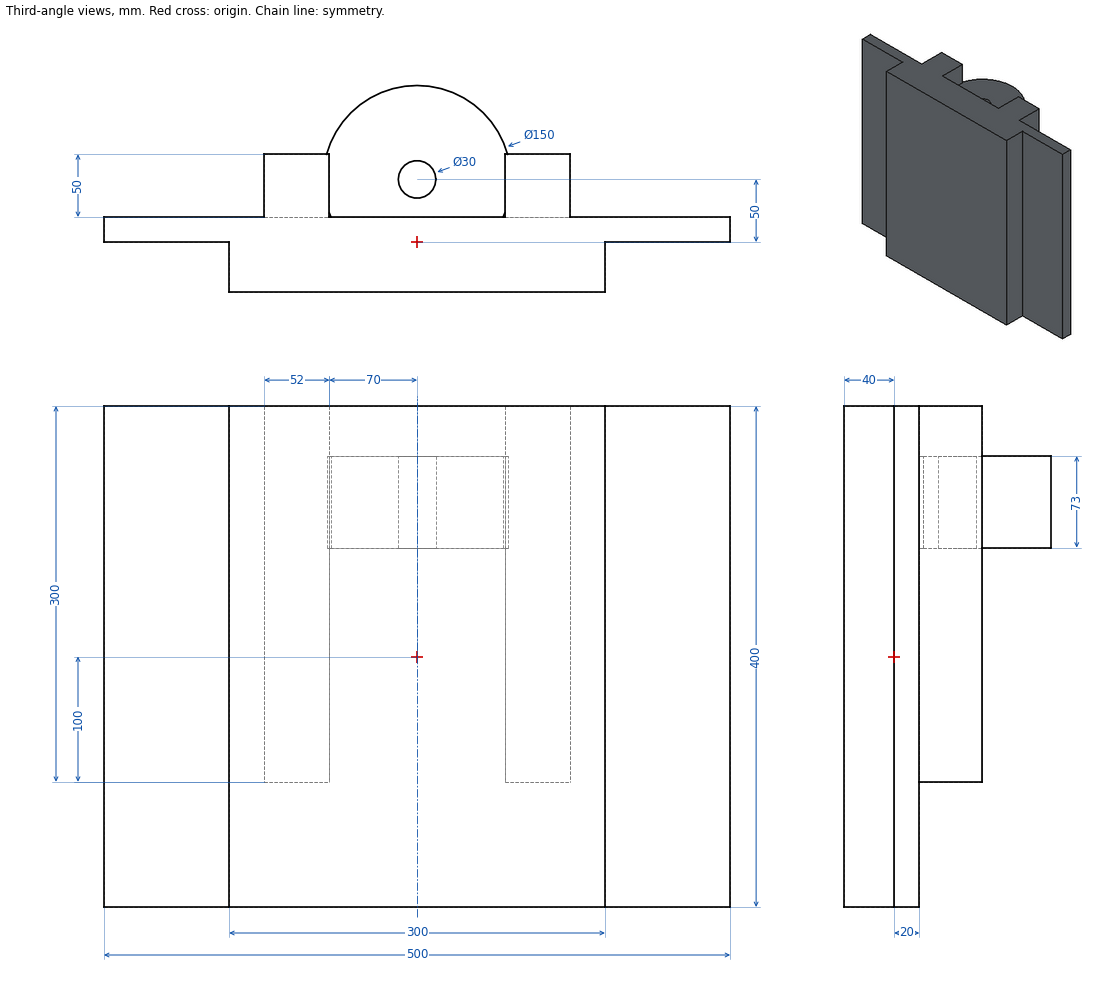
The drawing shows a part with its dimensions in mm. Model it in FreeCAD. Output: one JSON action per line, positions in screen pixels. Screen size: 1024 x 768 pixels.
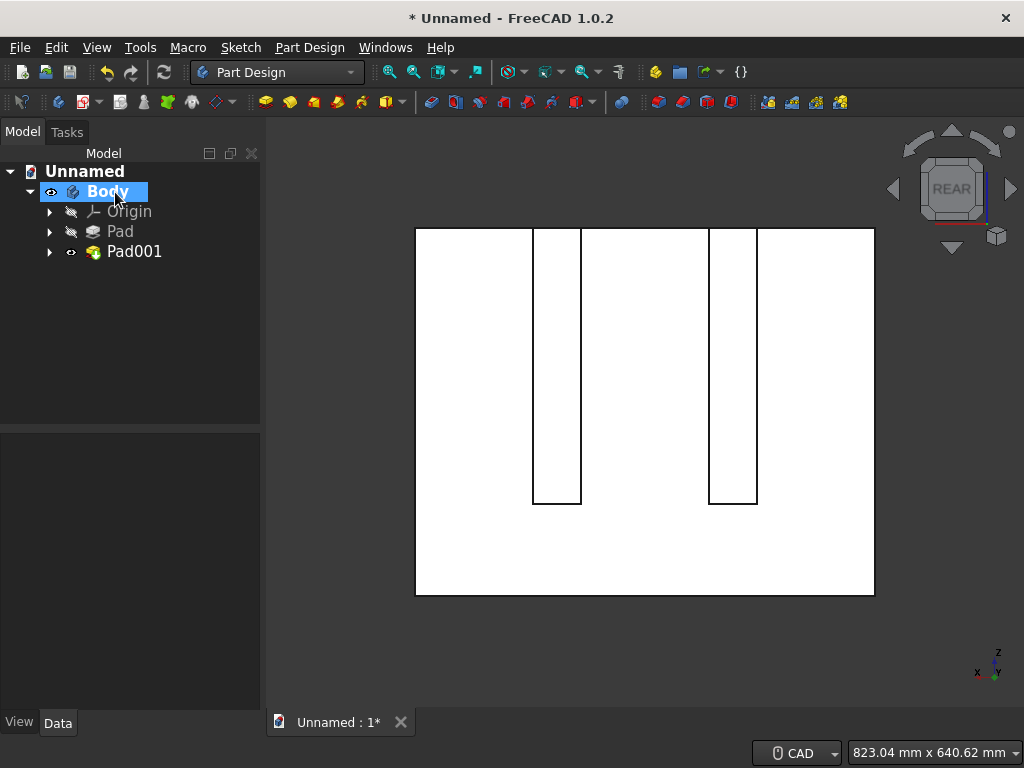
{"action": "left_click", "coordinate": [84, 102]}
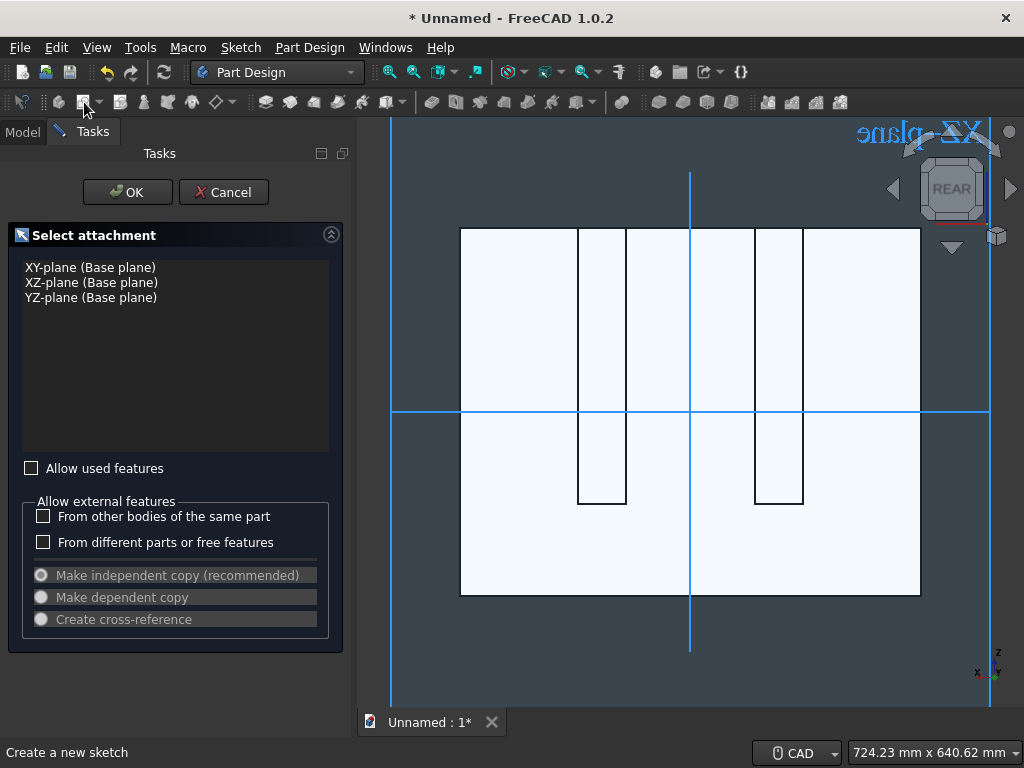
{"action": "left_click", "coordinate": [82, 282]}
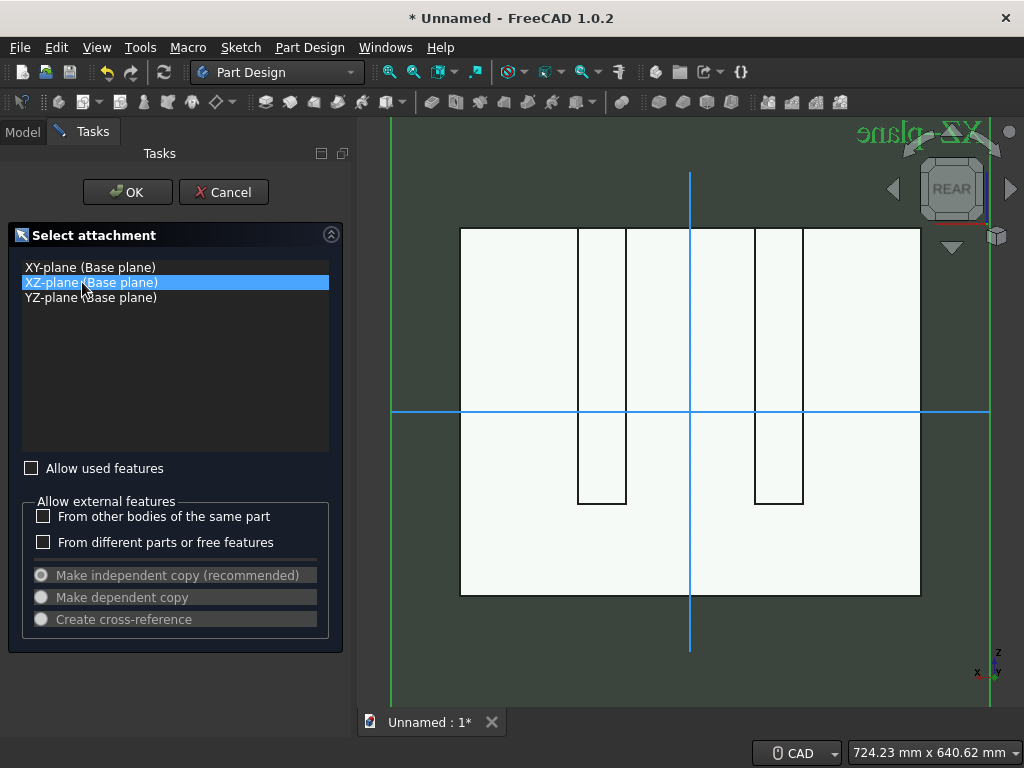
{"action": "left_click", "coordinate": [128, 192]}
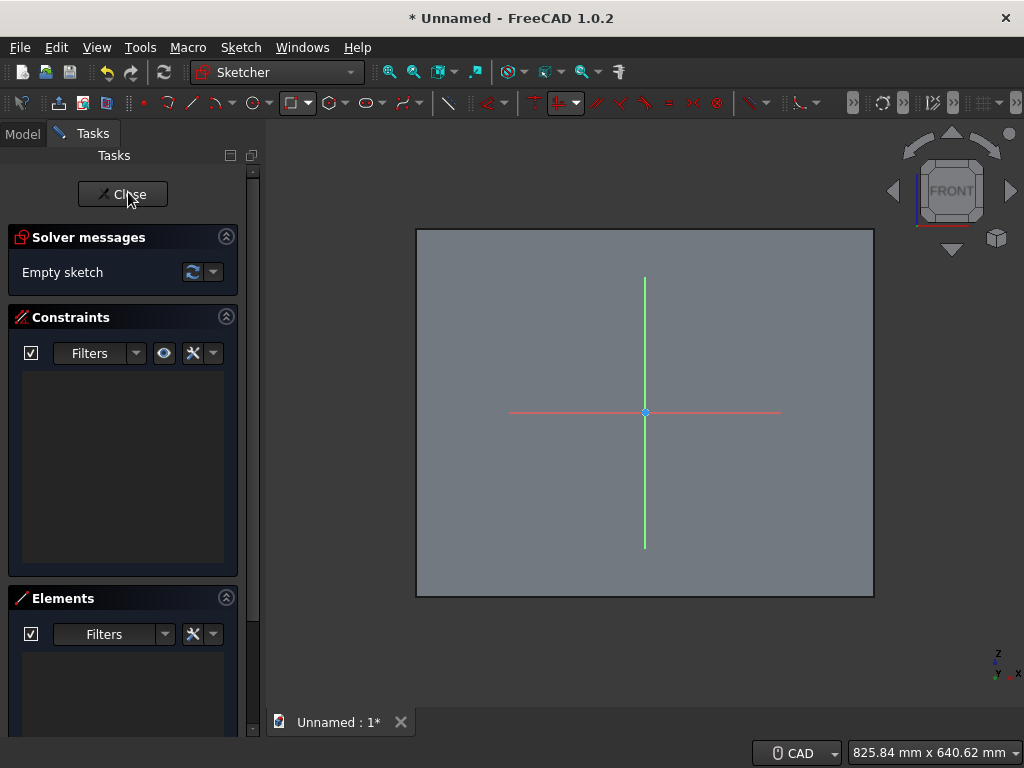
{"action": "key", "text": "g v"}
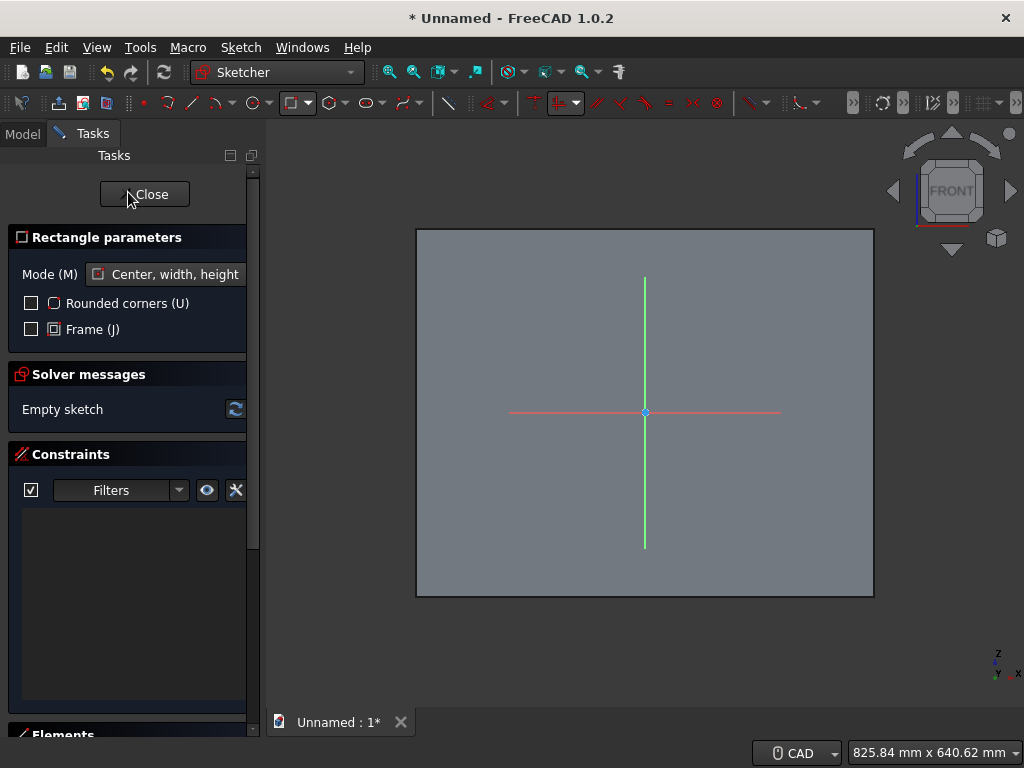
{"action": "left_click", "coordinate": [645, 413]}
{"action": "left_click", "coordinate": [783, 229]}
{"action": "key", "text": "Escape"}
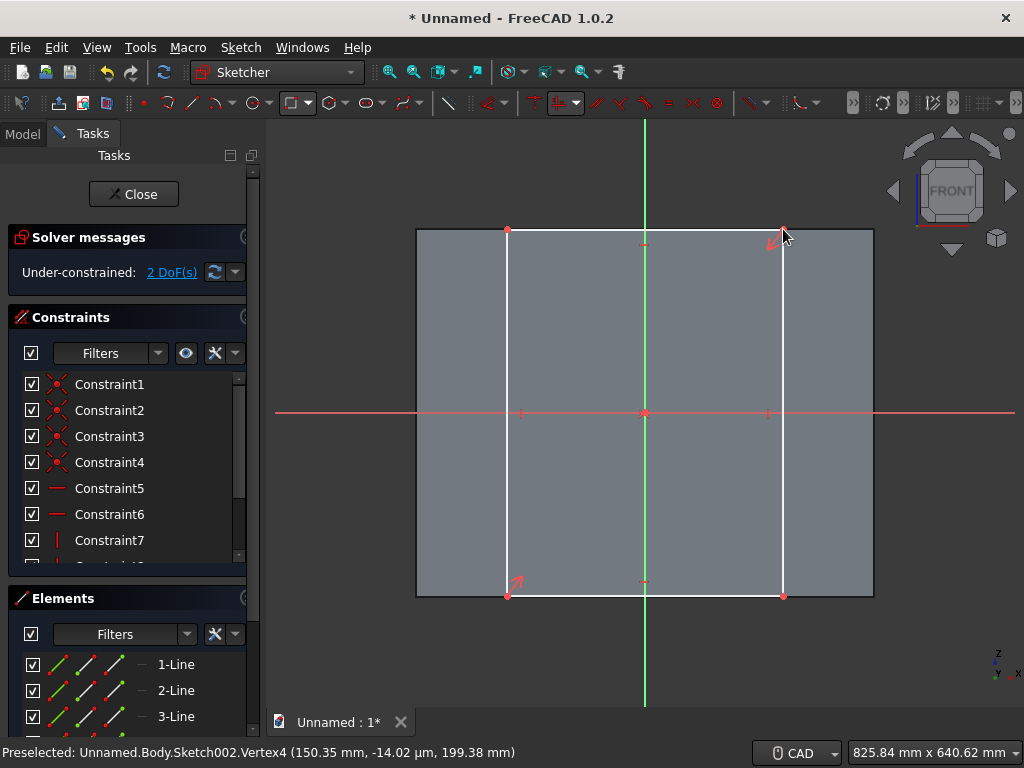
{"action": "key", "text": "d"}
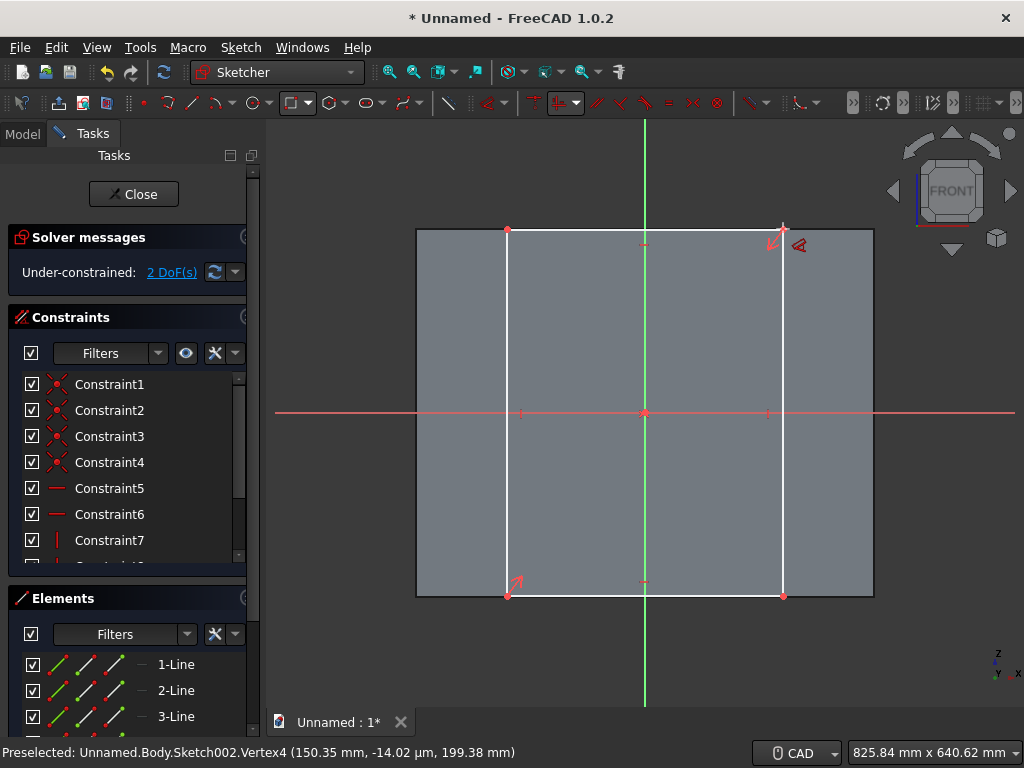
{"action": "left_click", "coordinate": [590, 596]}
{"action": "left_click", "coordinate": [582, 630]}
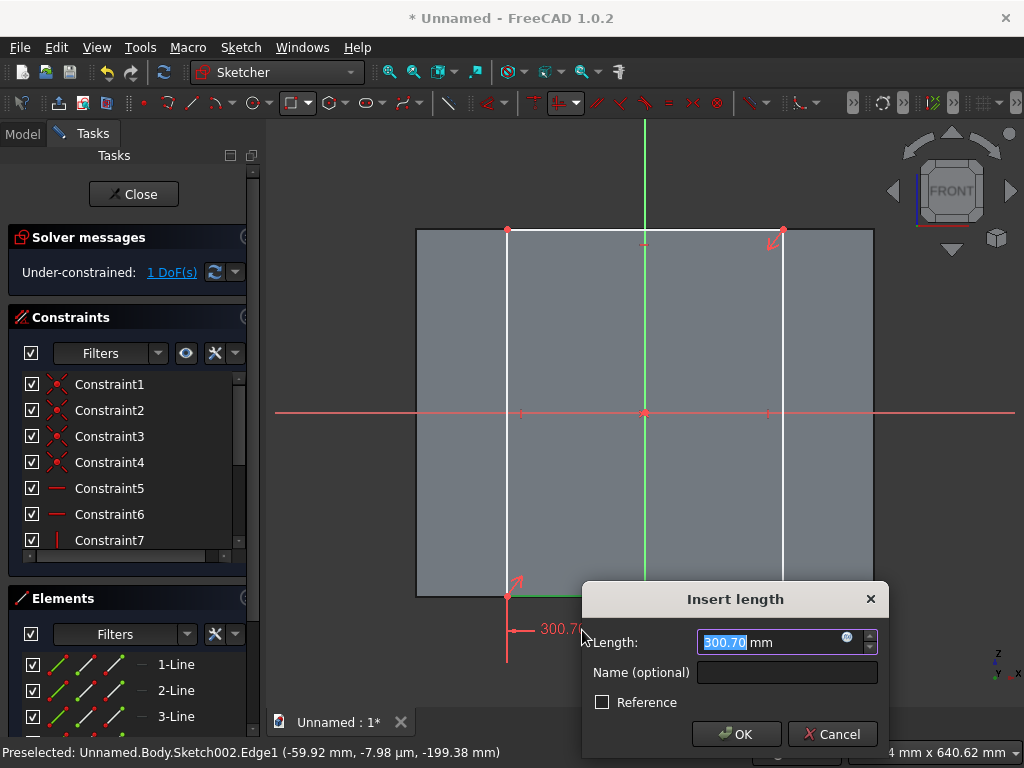
{"action": "type", "text": "300"}
{"action": "key", "text": "Return"}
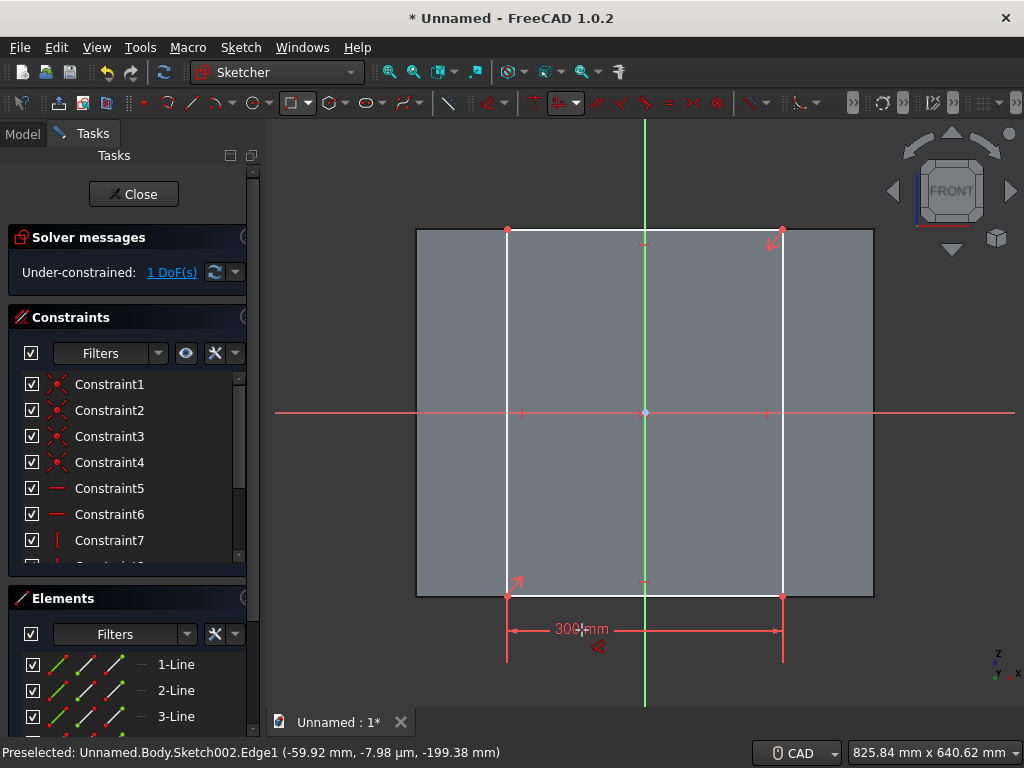
{"action": "left_click", "coordinate": [783, 486]}
{"action": "left_click", "coordinate": [817, 329]}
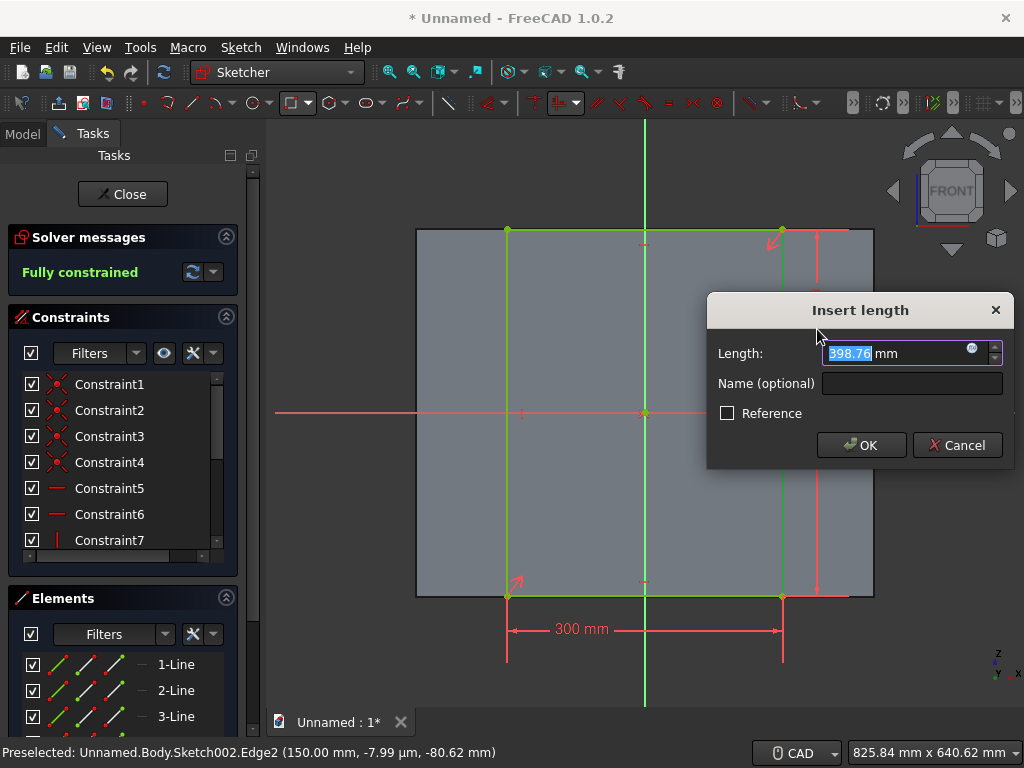
{"action": "type", "text": "400"}
{"action": "key", "text": "Return"}
{"action": "key", "text": "Escape"}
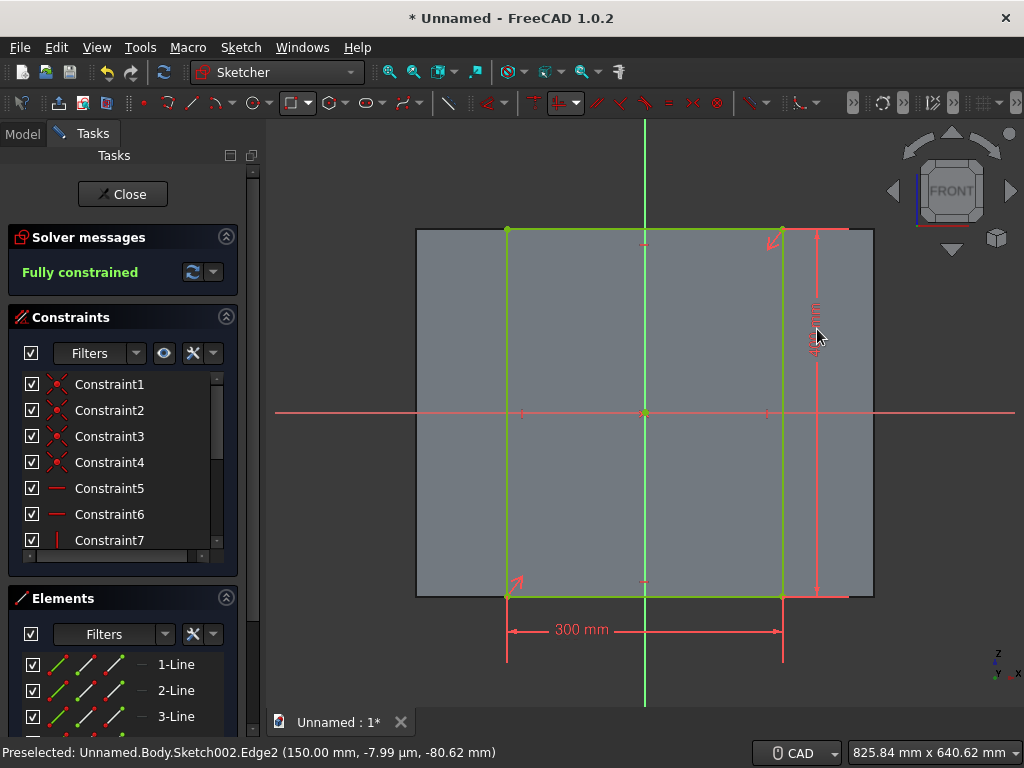
{"action": "left_click", "coordinate": [123, 194]}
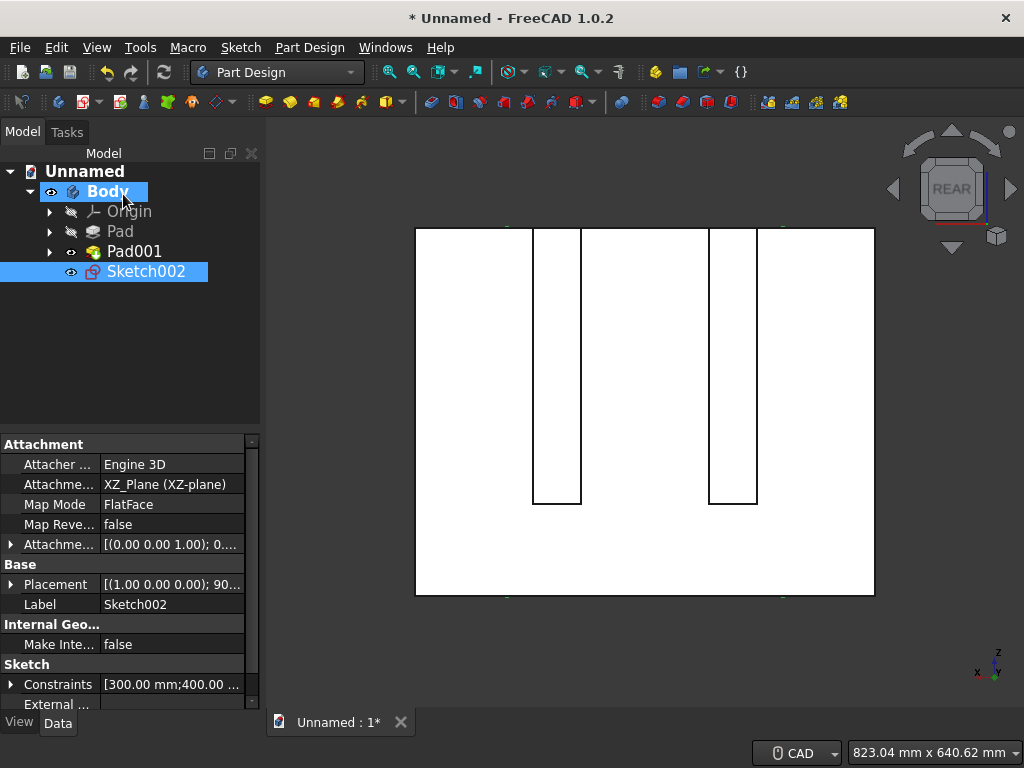
{"action": "left_click", "coordinate": [266, 102]}